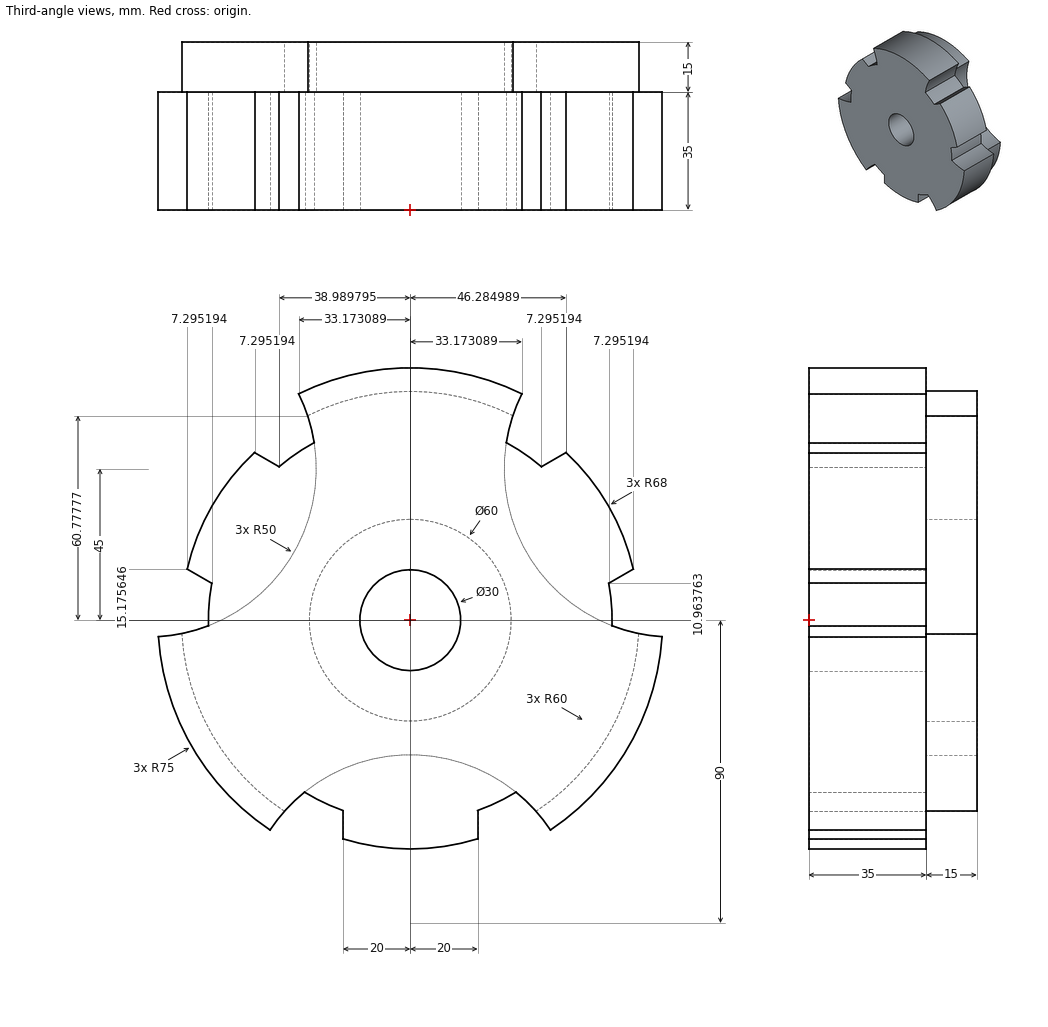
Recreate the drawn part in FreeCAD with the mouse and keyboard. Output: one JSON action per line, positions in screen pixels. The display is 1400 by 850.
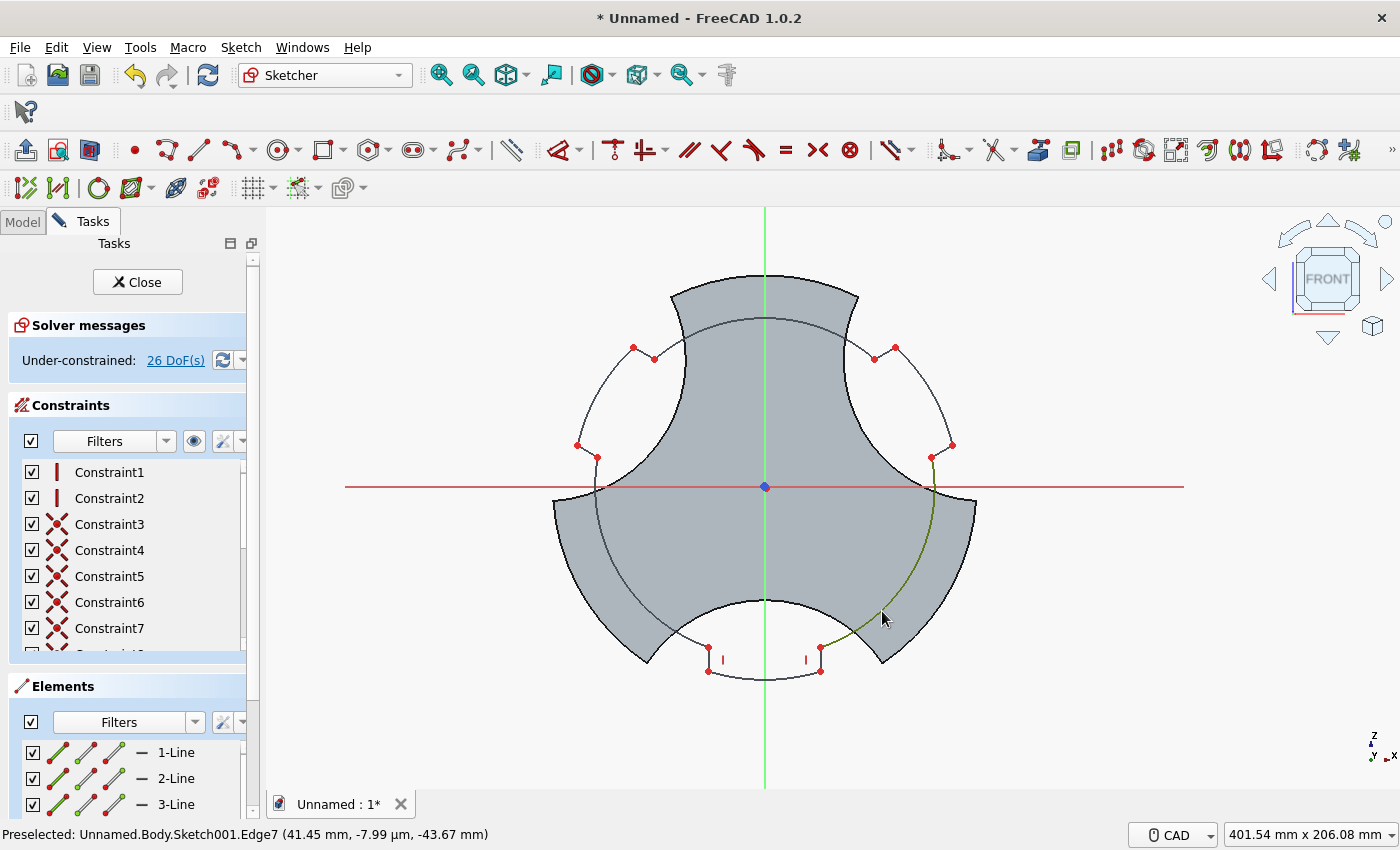
{"action": "left_click", "coordinate": [812, 325]}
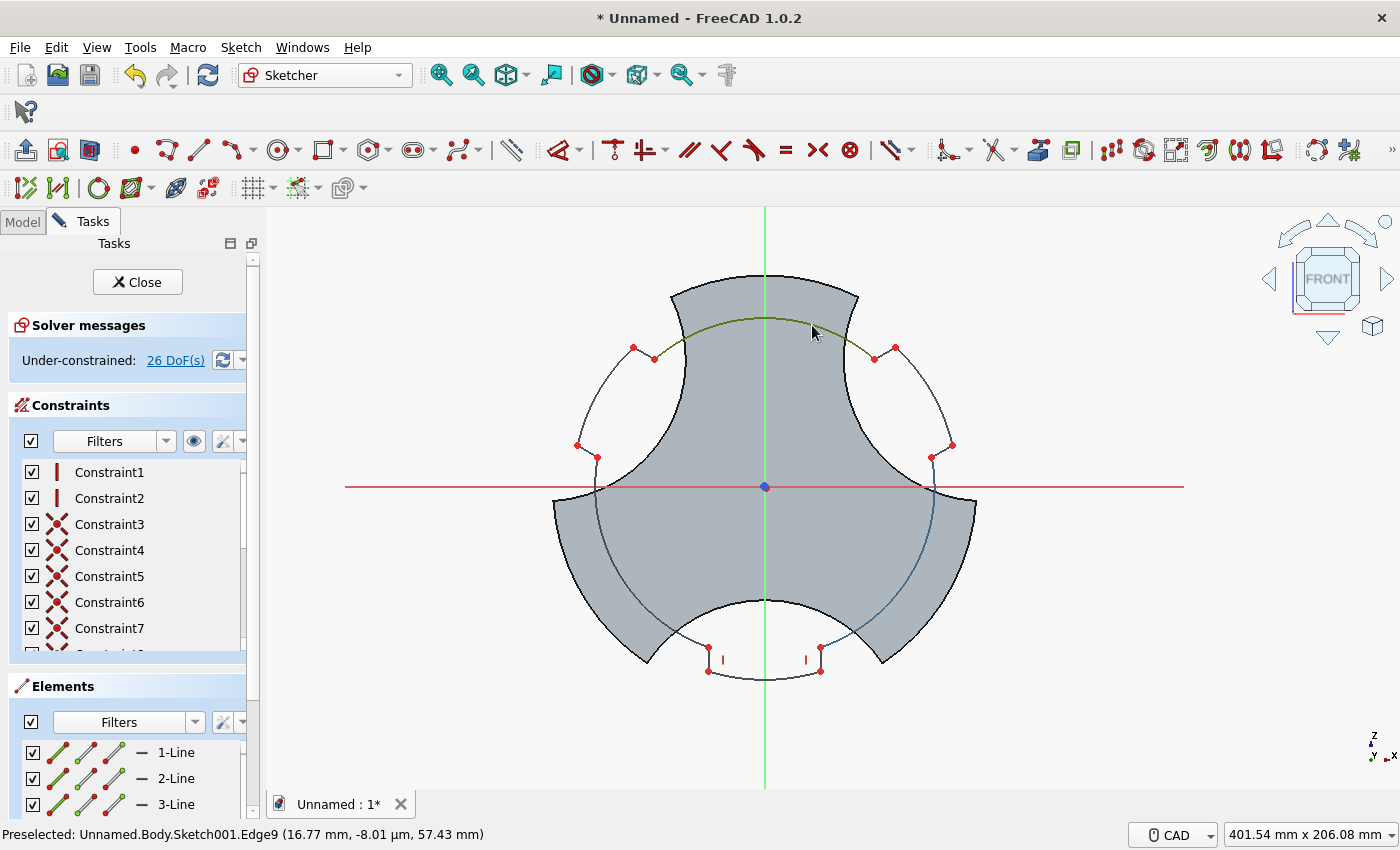
{"action": "left_click", "coordinate": [614, 150]}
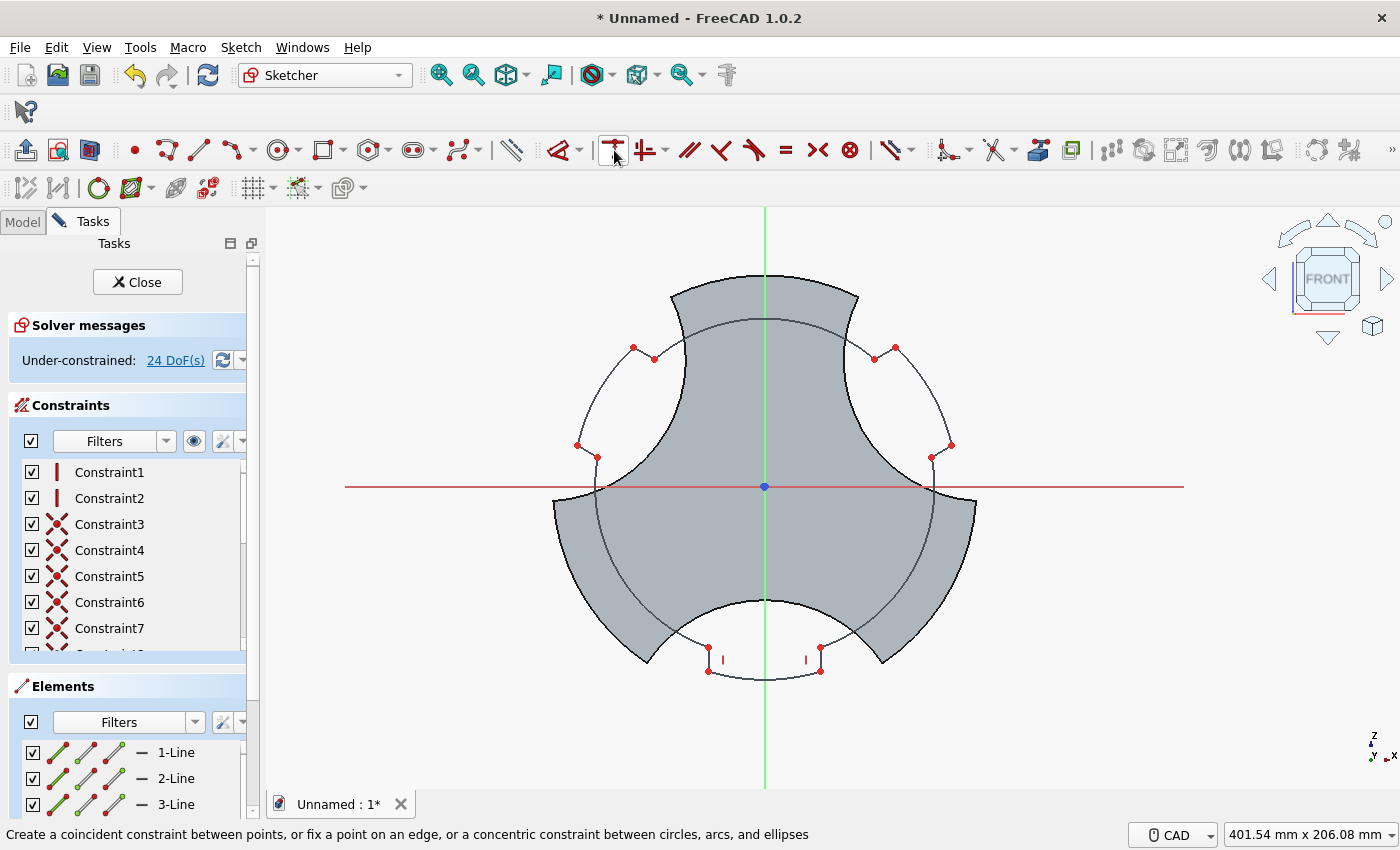
{"action": "left_click", "coordinate": [882, 610]}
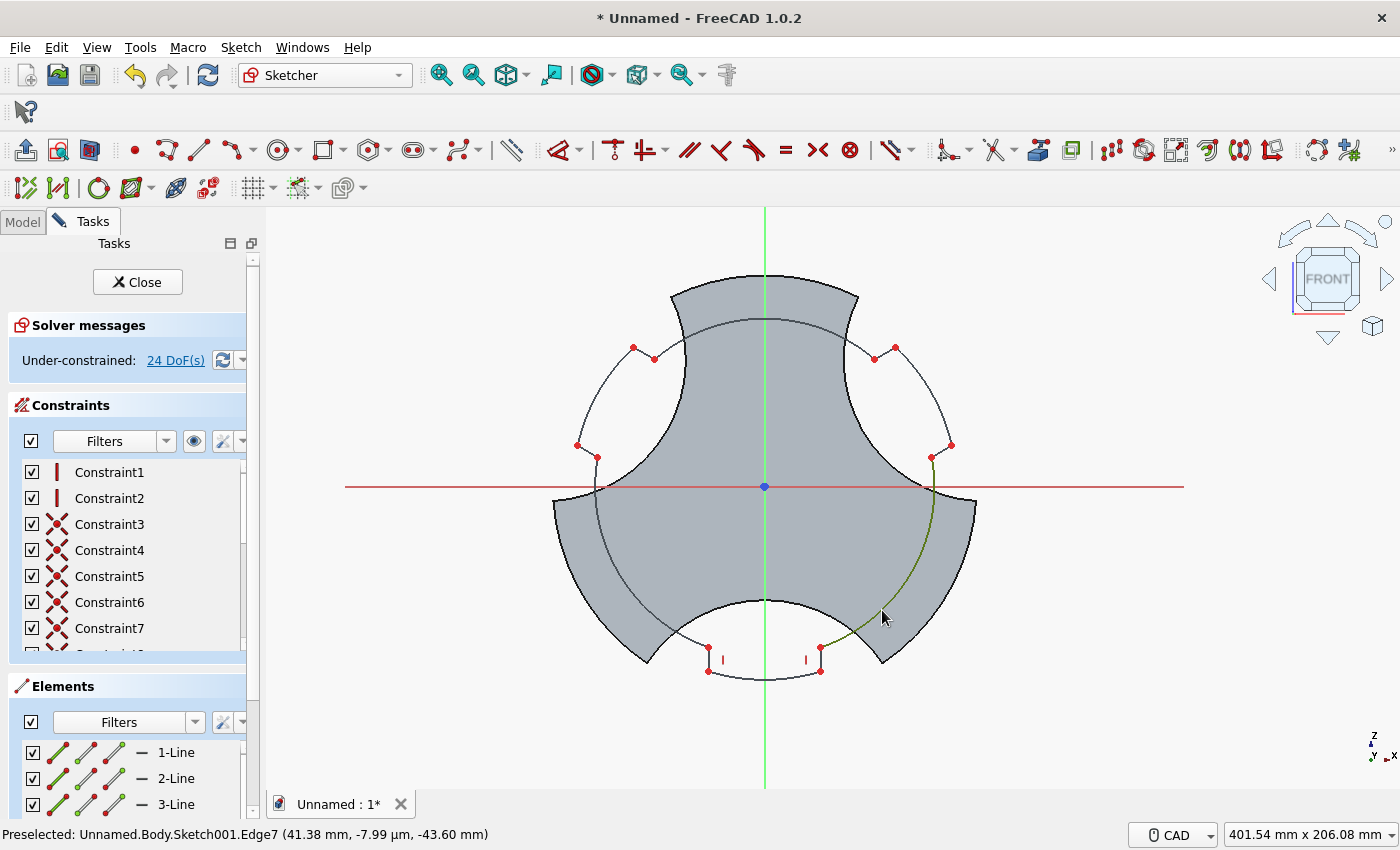
{"action": "left_click", "coordinate": [611, 373]}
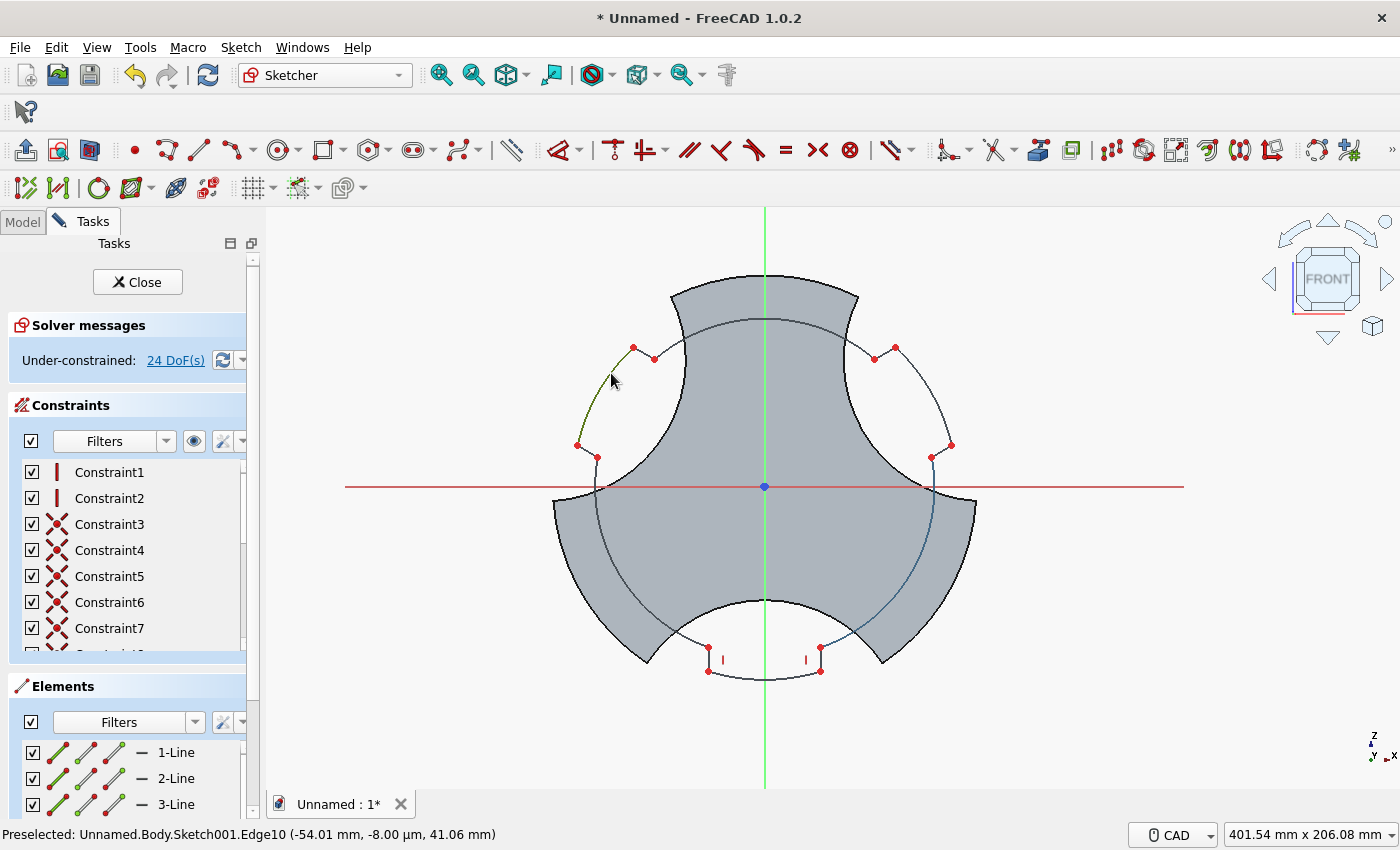
{"action": "left_click", "coordinate": [614, 150]}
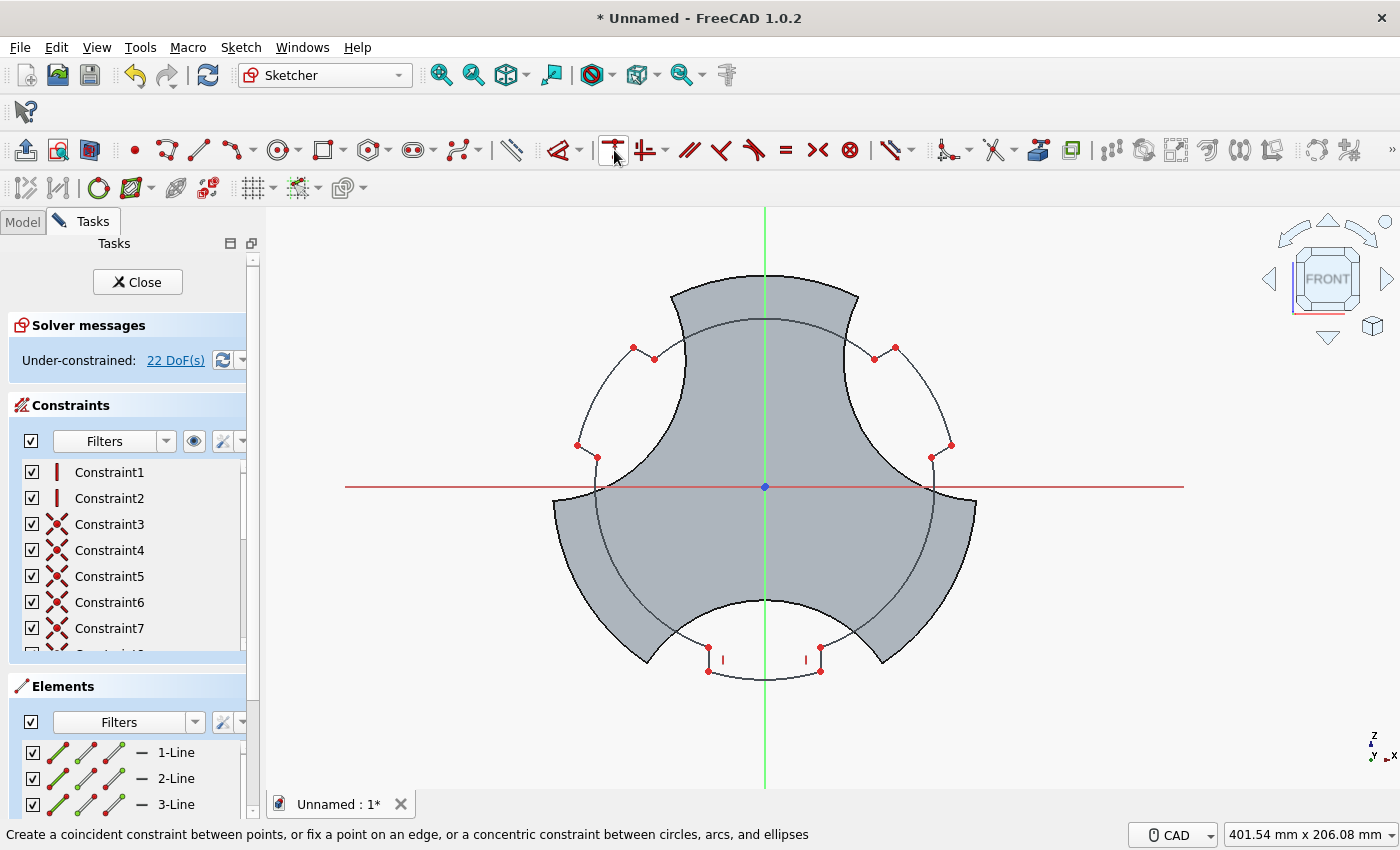
{"action": "left_click", "coordinate": [882, 610]}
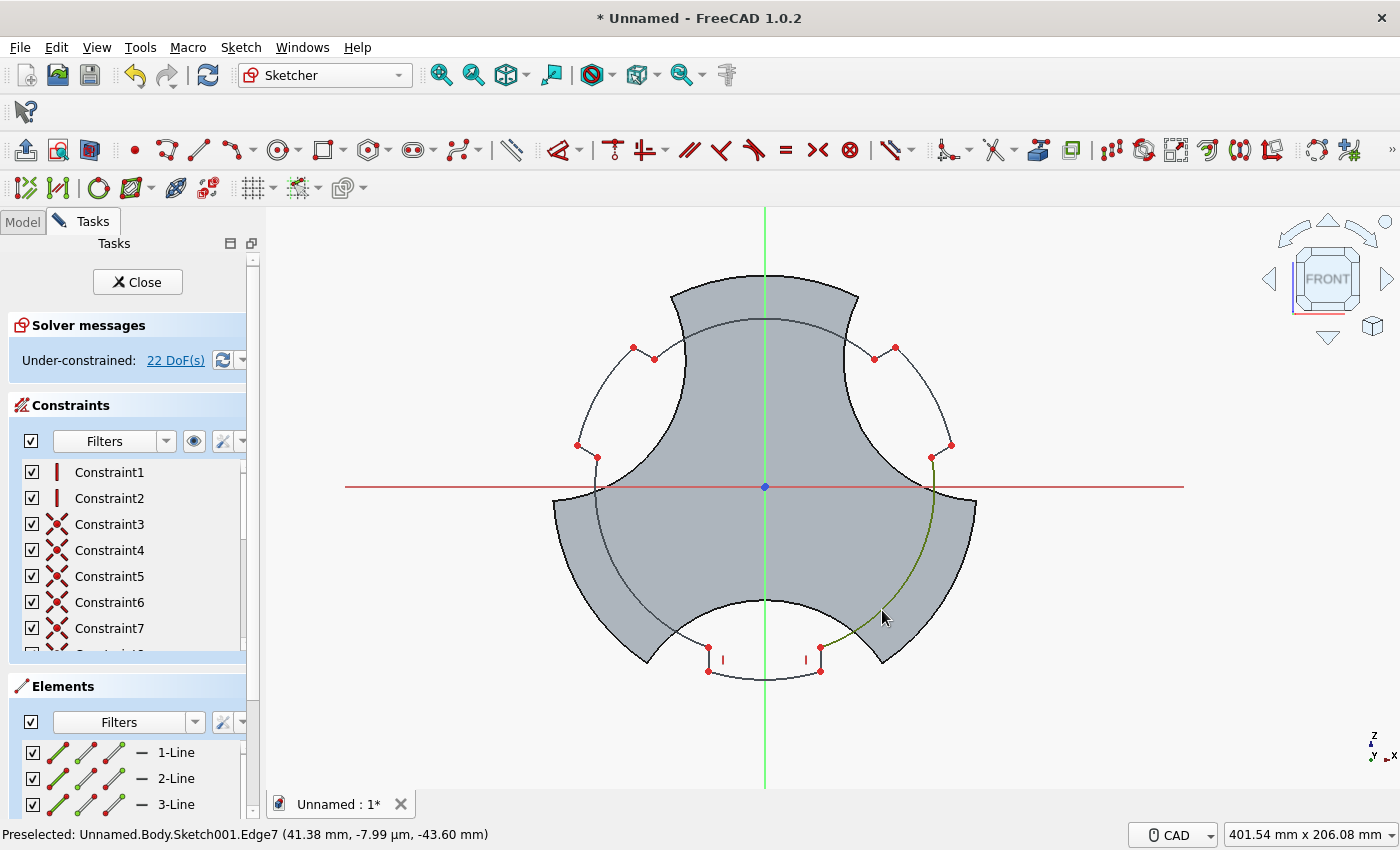
{"action": "left_click", "coordinate": [600, 529]}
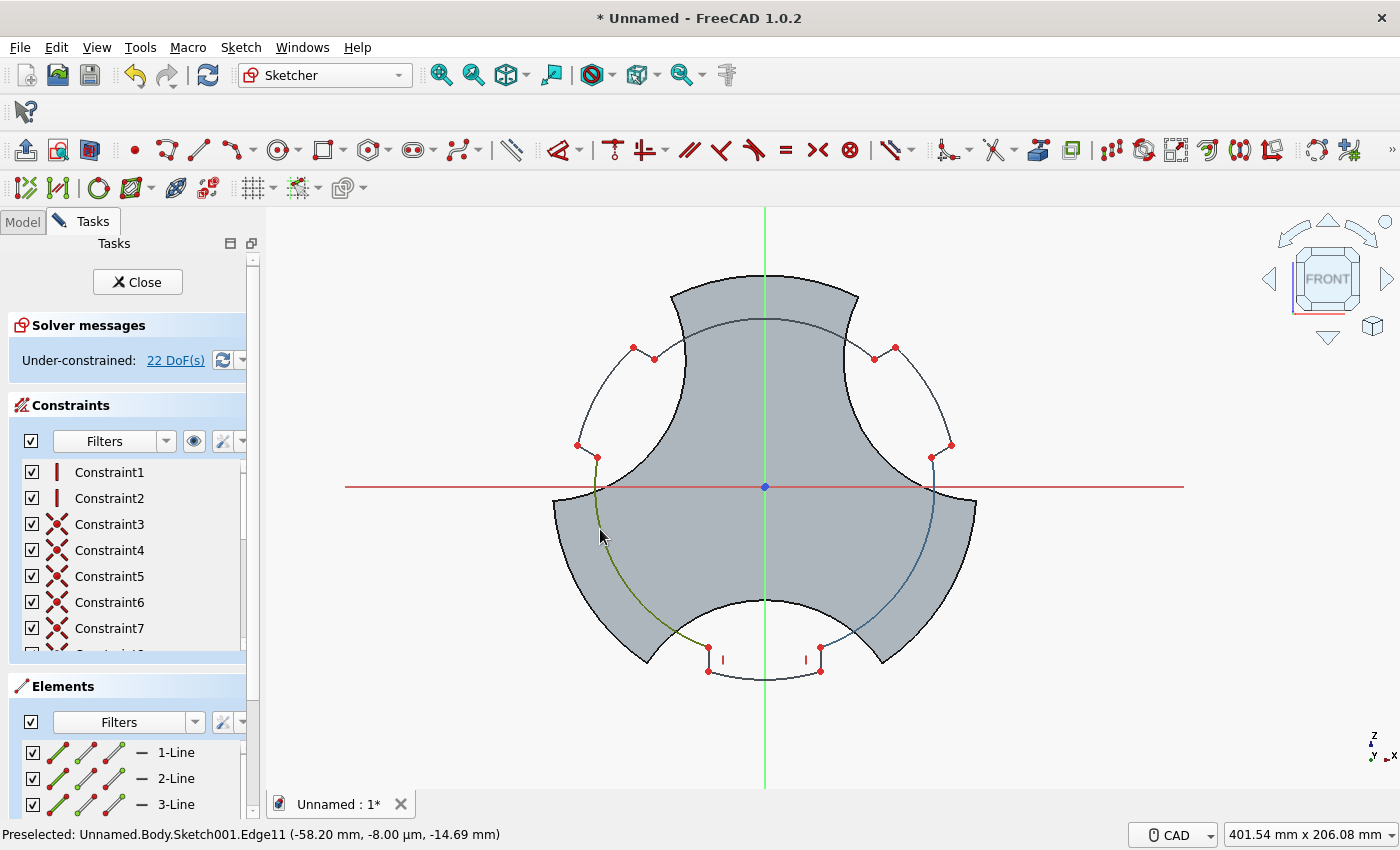
{"action": "left_click", "coordinate": [614, 150]}